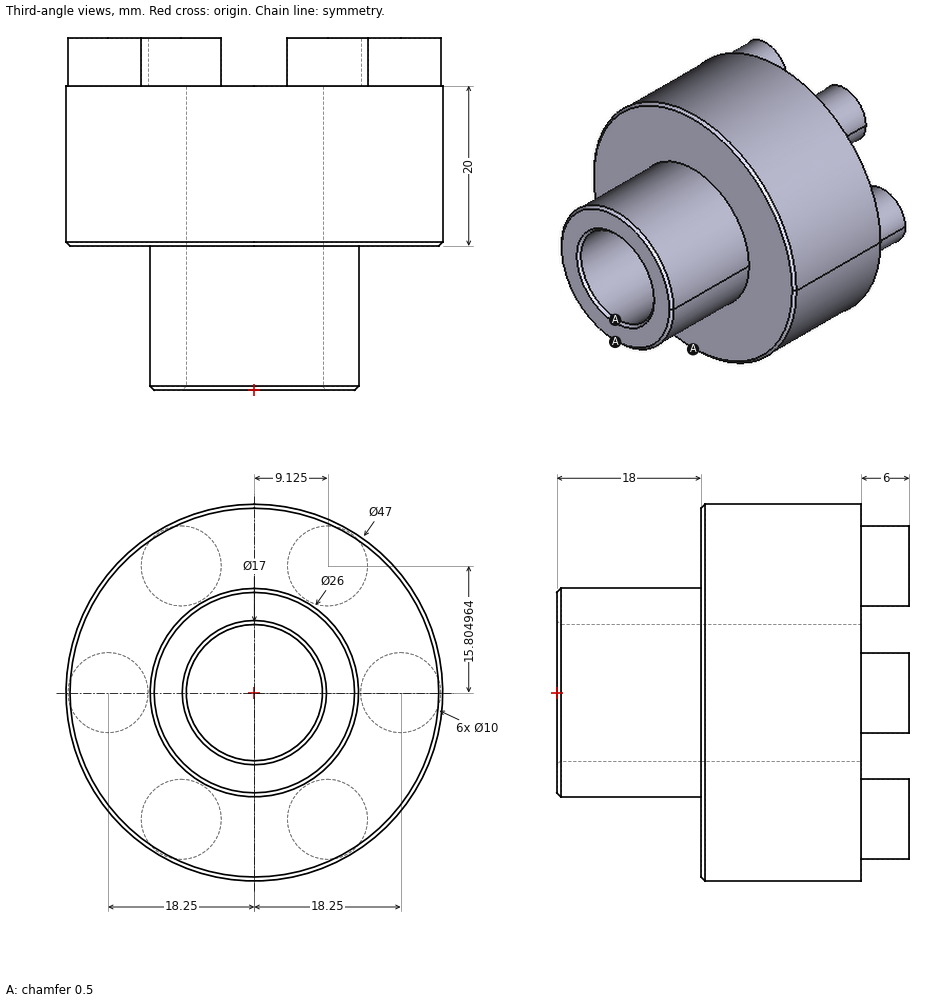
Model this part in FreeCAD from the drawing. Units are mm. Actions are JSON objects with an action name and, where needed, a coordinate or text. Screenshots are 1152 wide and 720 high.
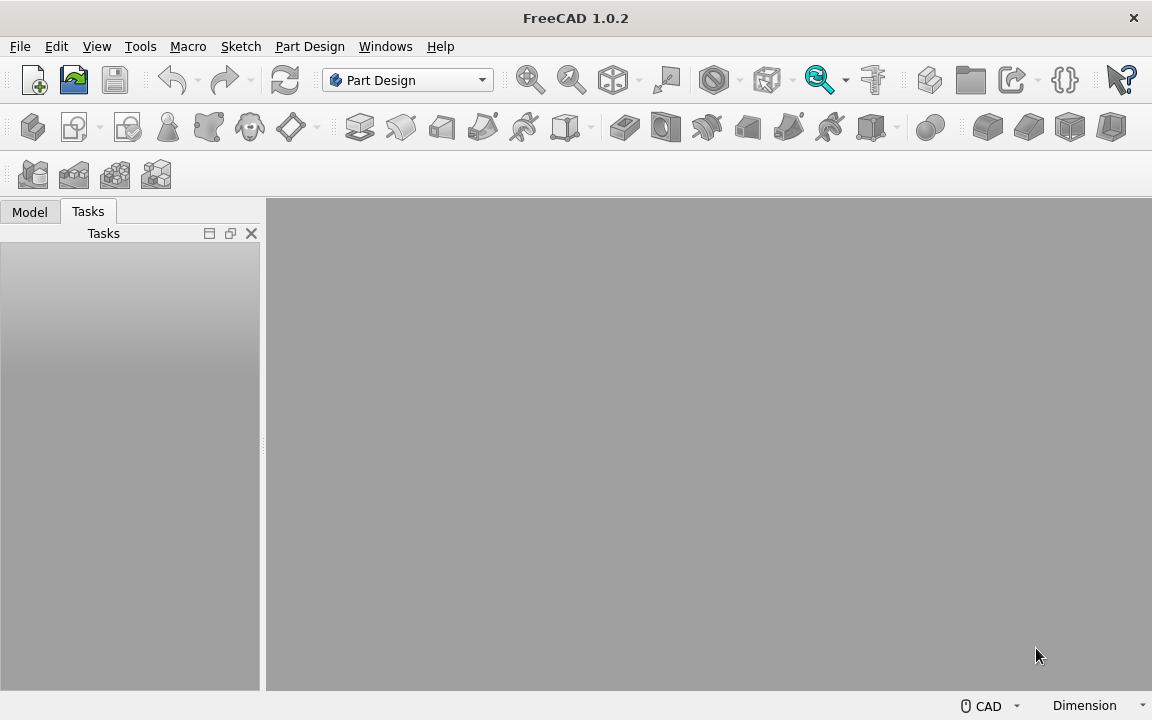
{"action": "left_click", "coordinate": [33, 80]}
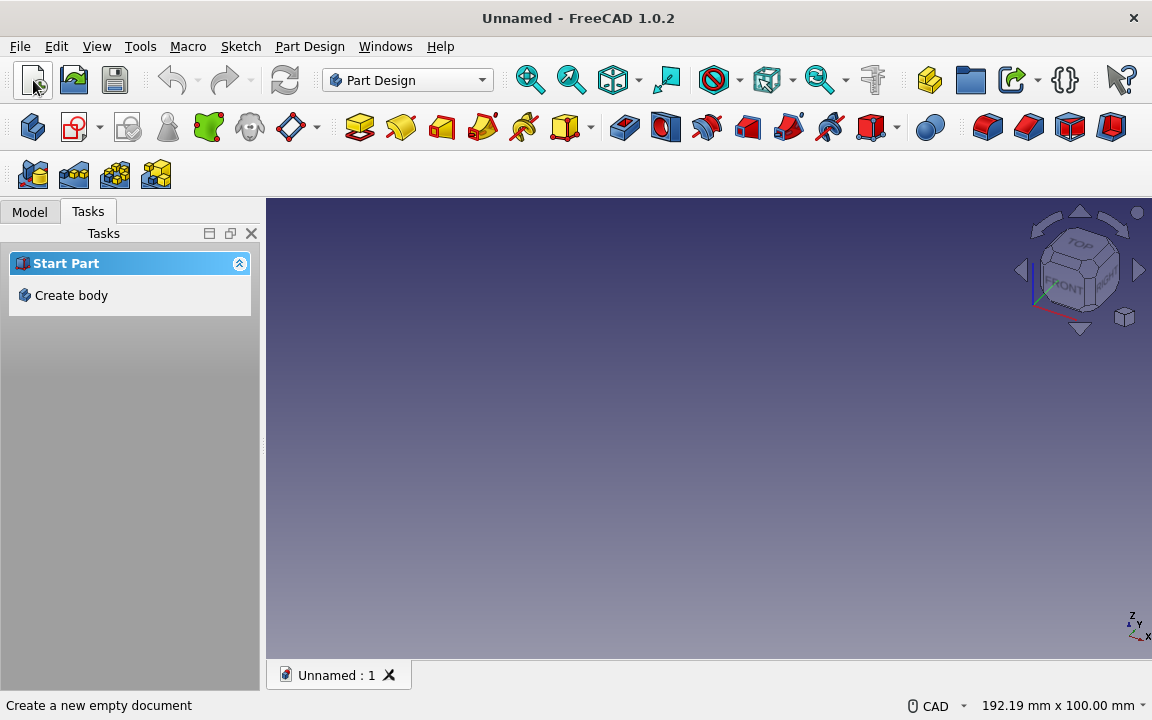
{"action": "left_click", "coordinate": [74, 128]}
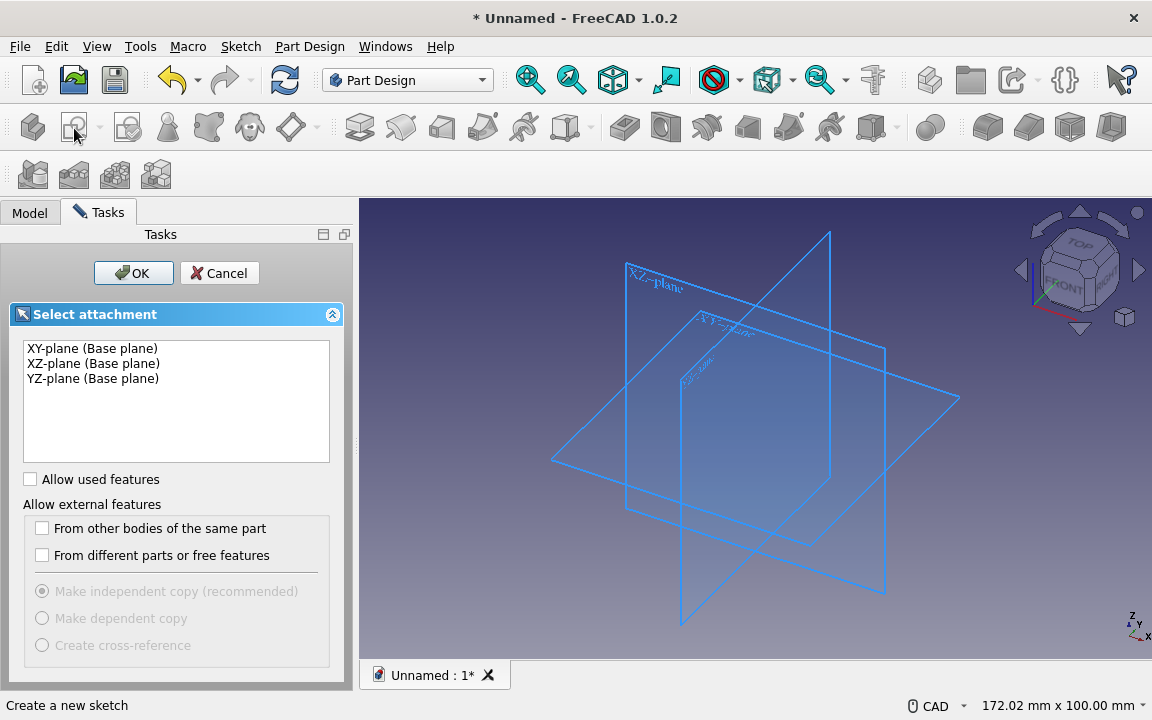
{"action": "left_click", "coordinate": [84, 364]}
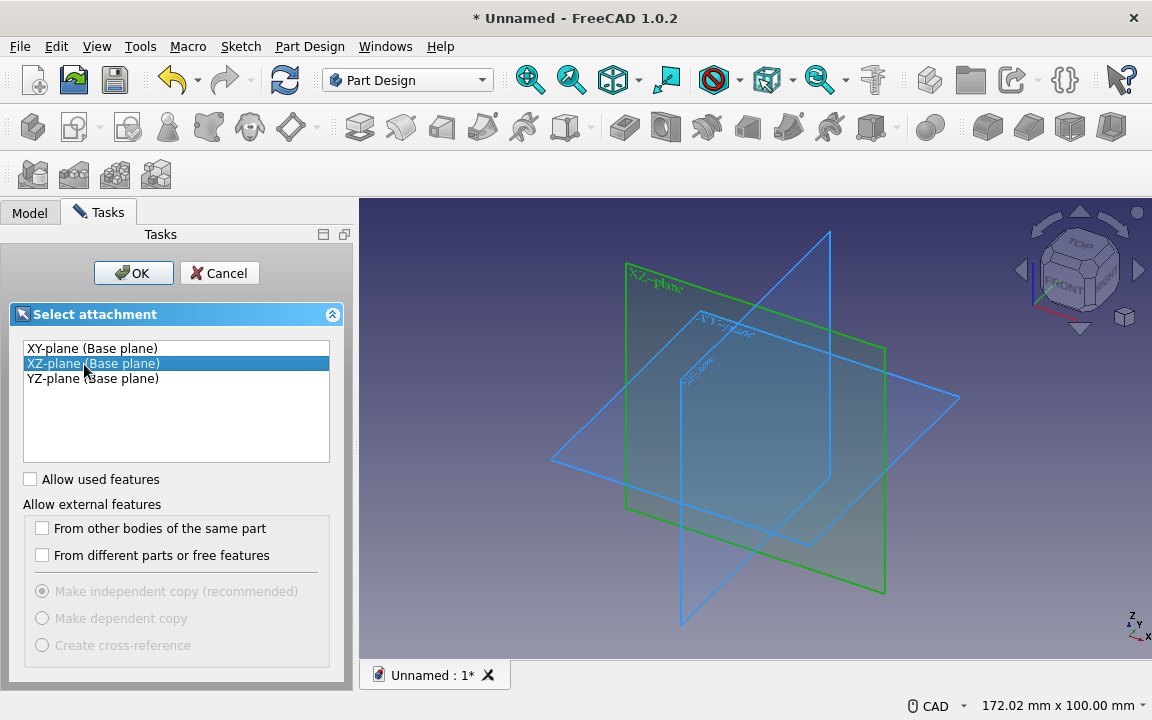
{"action": "left_click", "coordinate": [134, 273]}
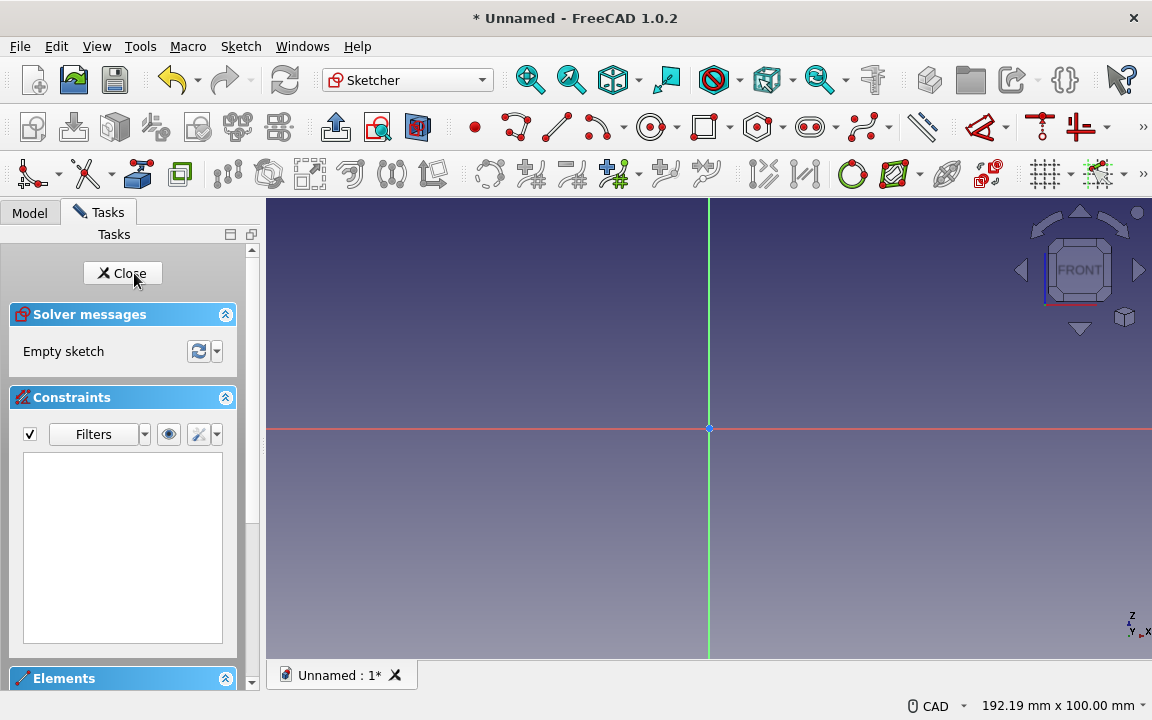
{"action": "scroll", "coordinate": [765, 428], "scroll_direction": "up", "scroll_amount": 4}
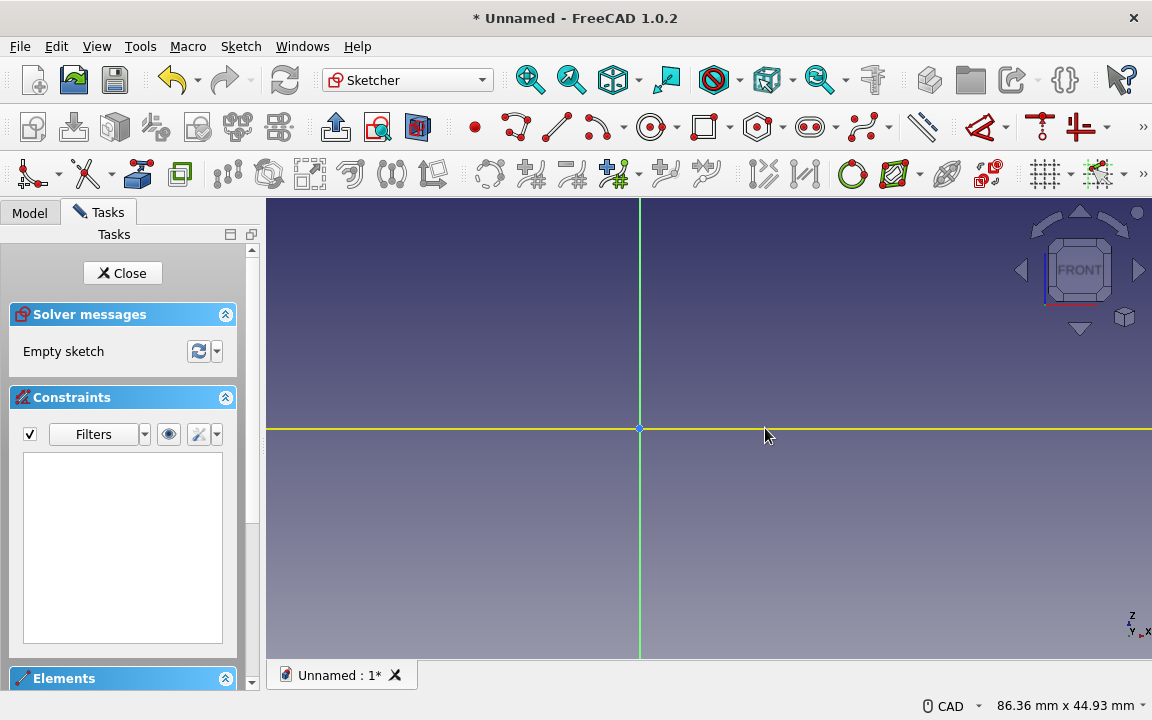
{"action": "left_click", "coordinate": [650, 128]}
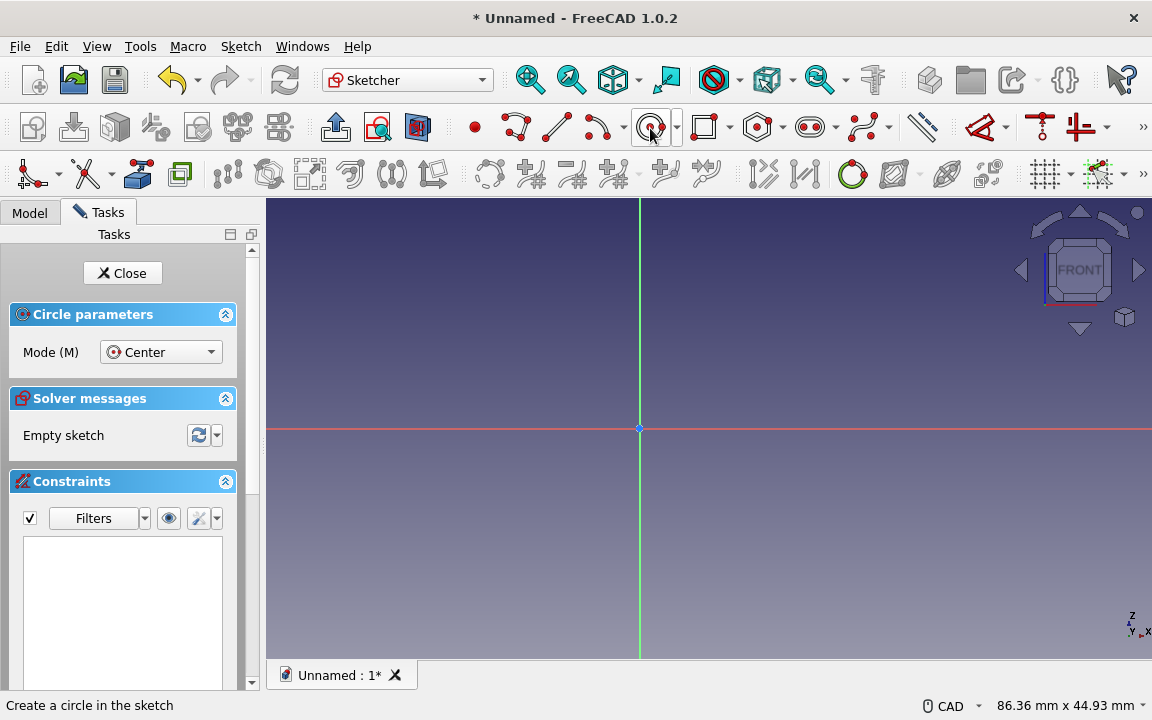
{"action": "left_click", "coordinate": [640, 428]}
{"action": "left_click", "coordinate": [734, 334]}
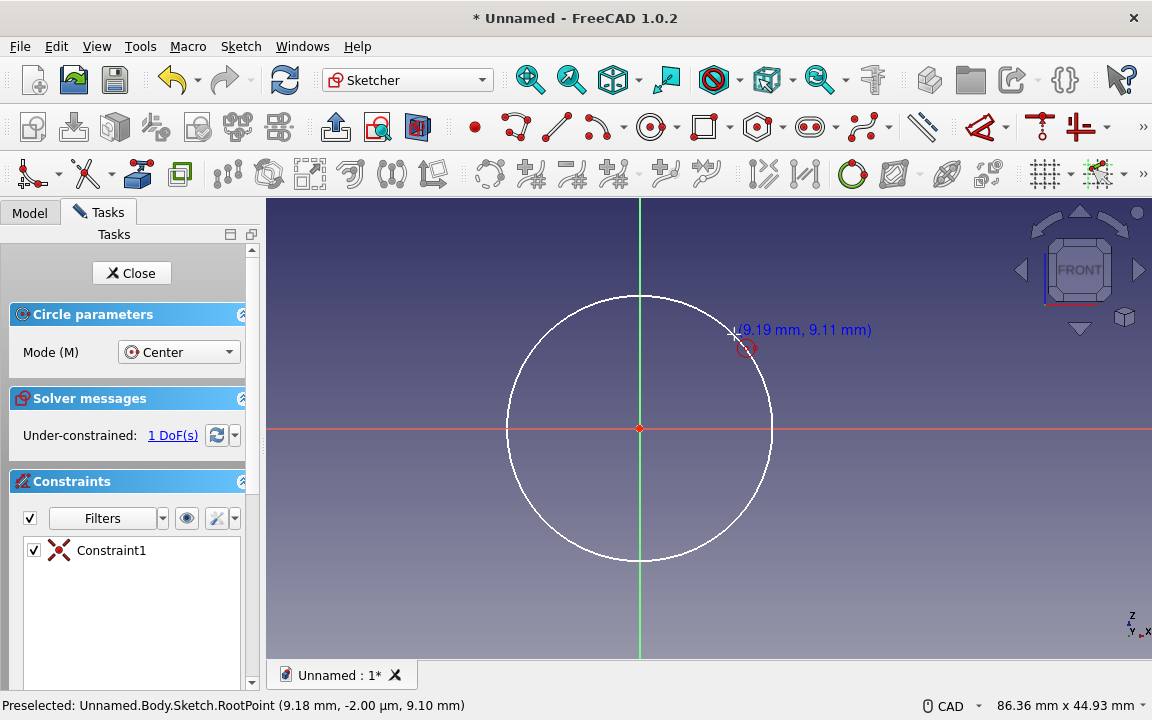
{"action": "left_click", "coordinate": [640, 428]}
{"action": "left_click", "coordinate": [701, 367]}
{"action": "key", "text": "Escape"}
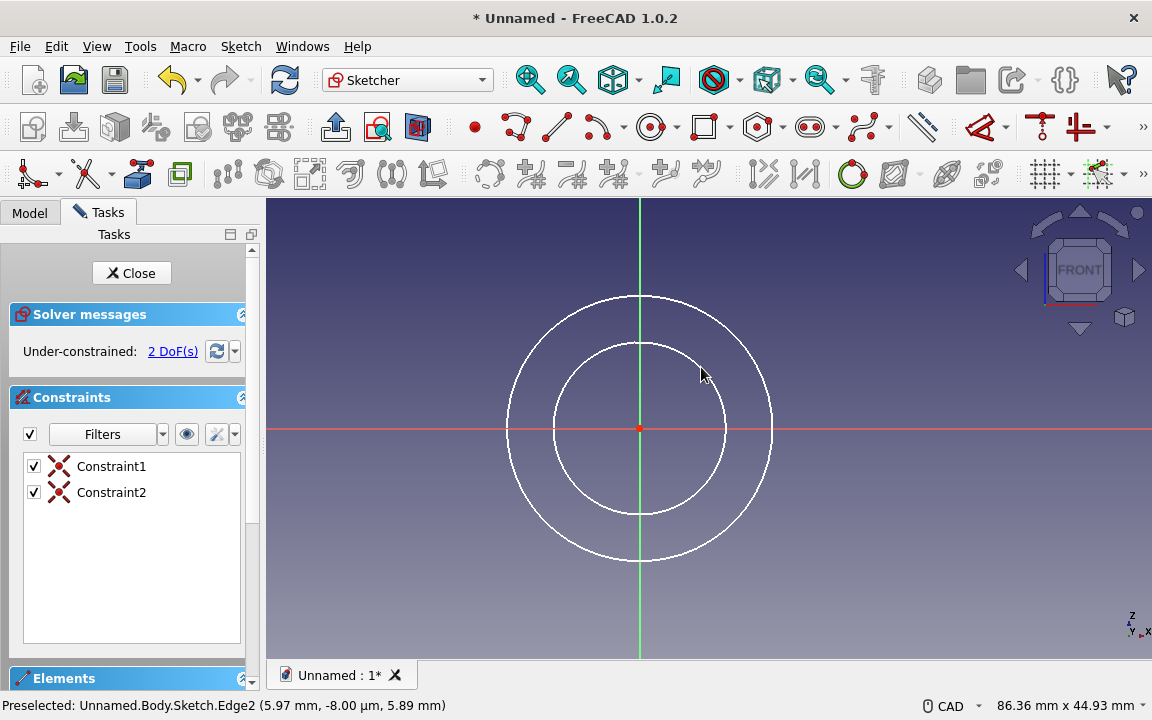
{"action": "left_click", "coordinate": [980, 128]}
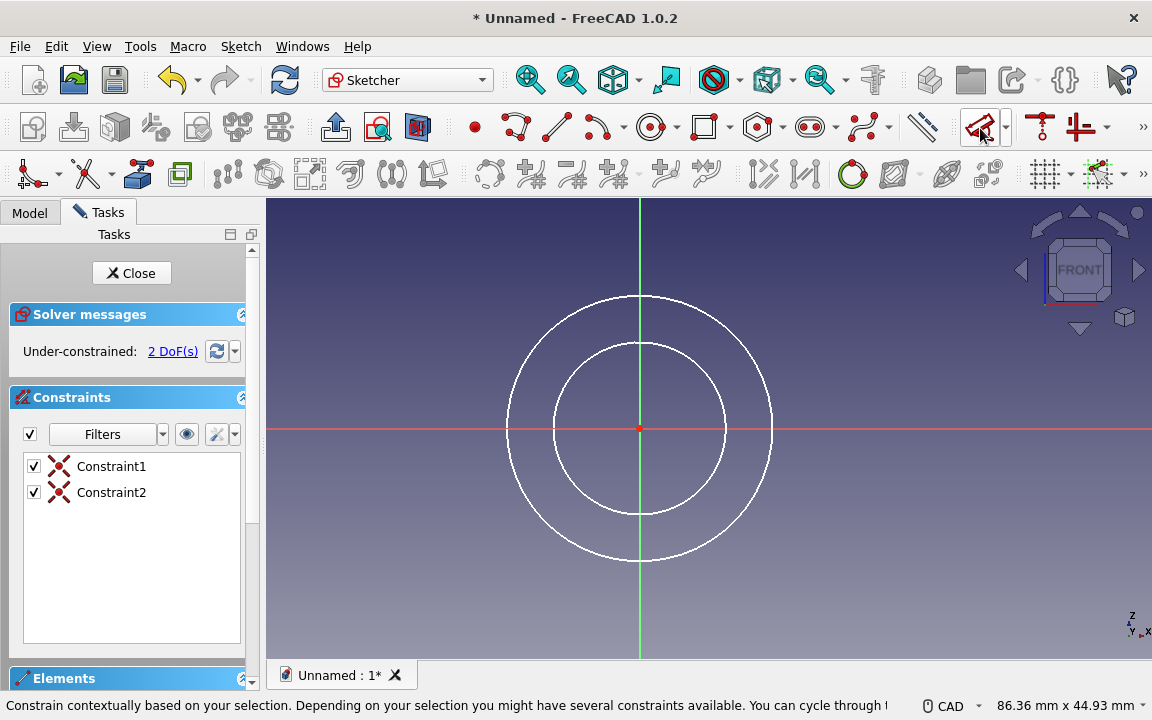
{"action": "left_click", "coordinate": [733, 334]}
{"action": "left_click", "coordinate": [755, 311]}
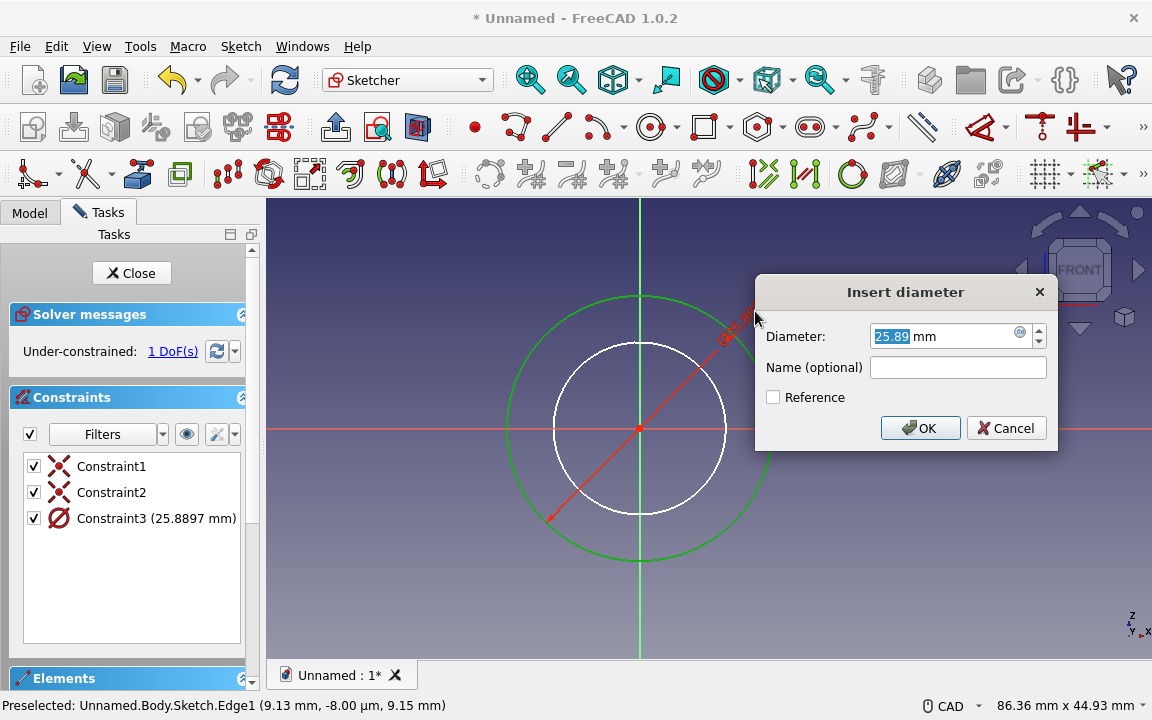
{"action": "type", "text": "26"}
{"action": "key", "text": "Return"}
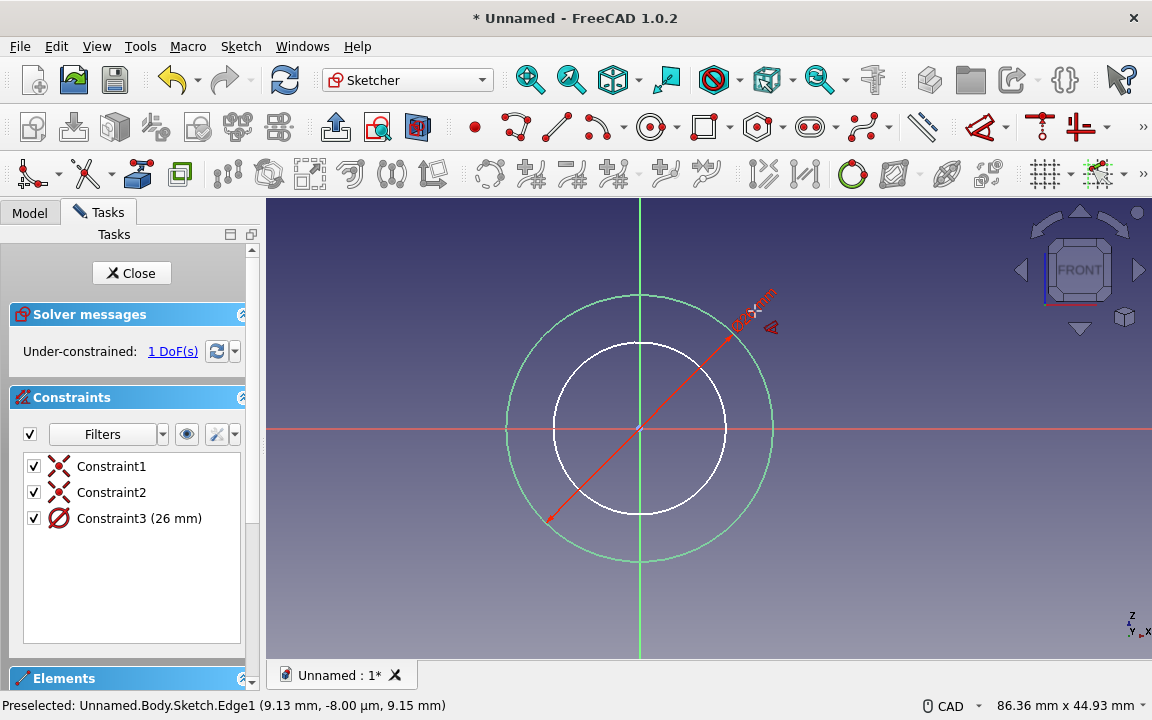
{"action": "left_click", "coordinate": [700, 367]}
{"action": "left_click", "coordinate": [722, 344]}